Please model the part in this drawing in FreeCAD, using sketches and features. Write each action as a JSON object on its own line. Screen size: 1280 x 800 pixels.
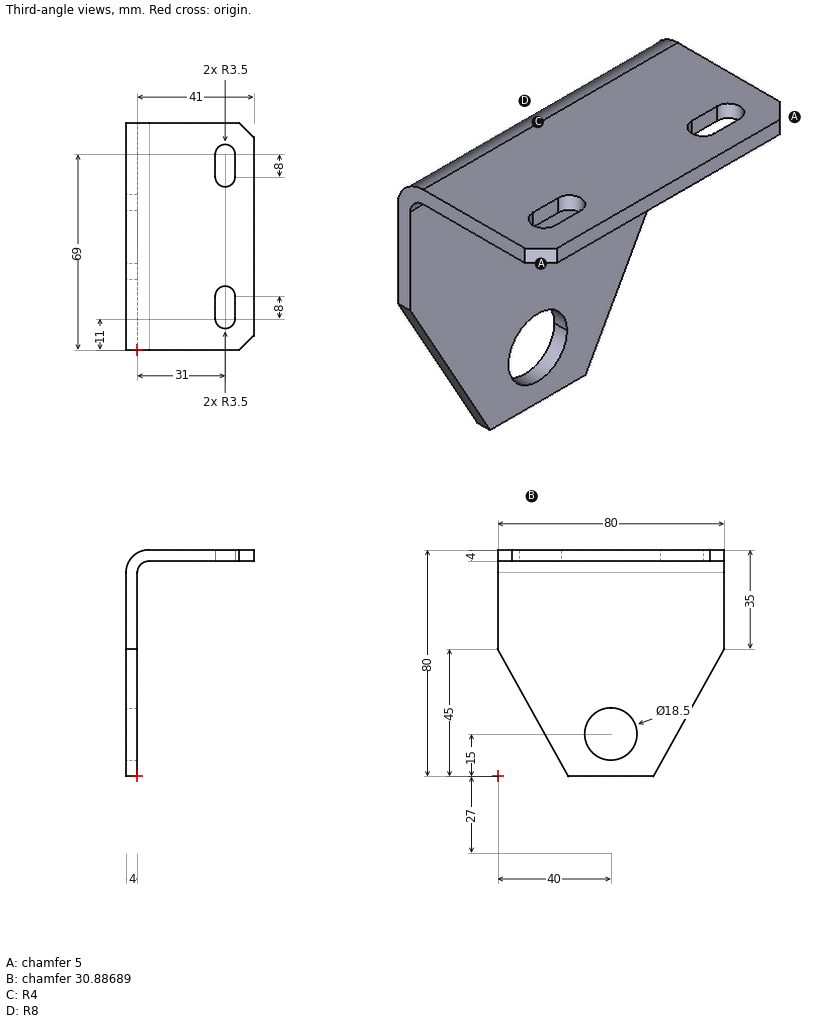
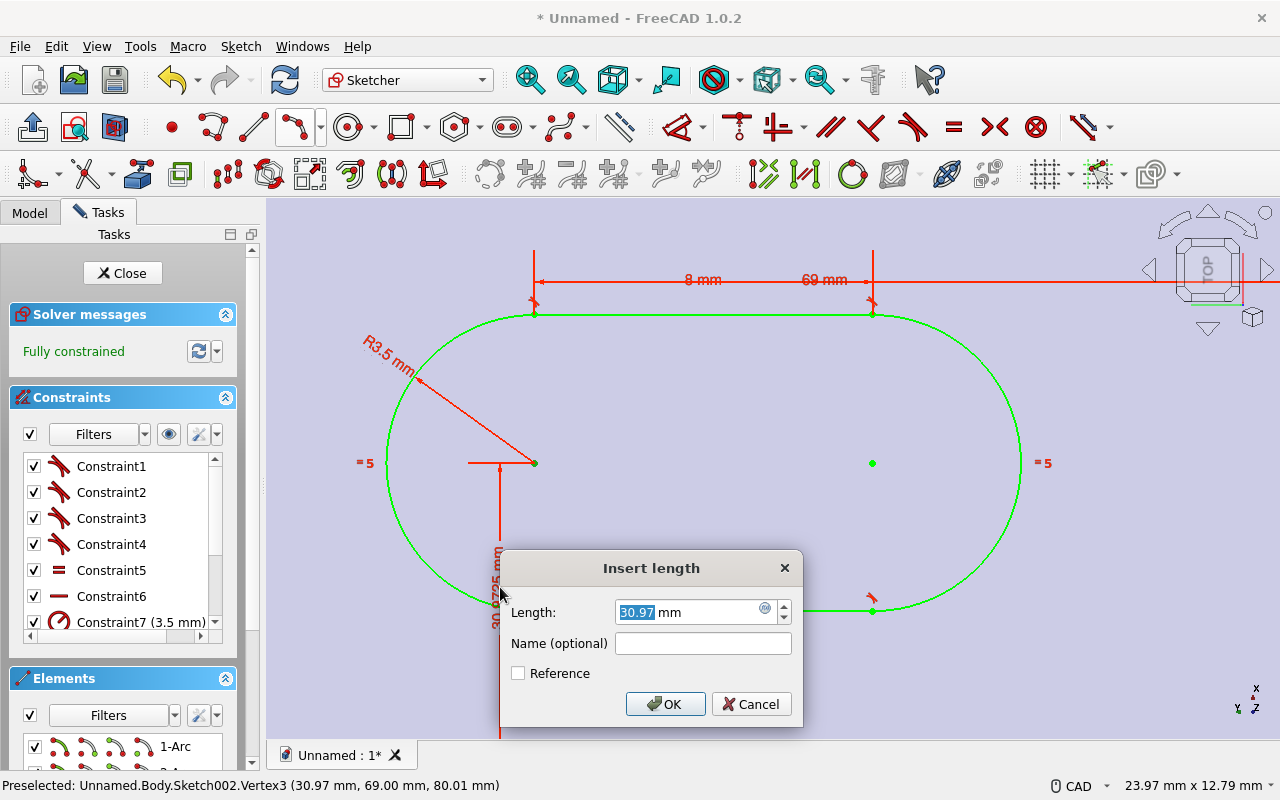
{"action": "type", "text": "31"}
{"action": "key", "text": "Return"}
{"action": "key", "text": "Escape"}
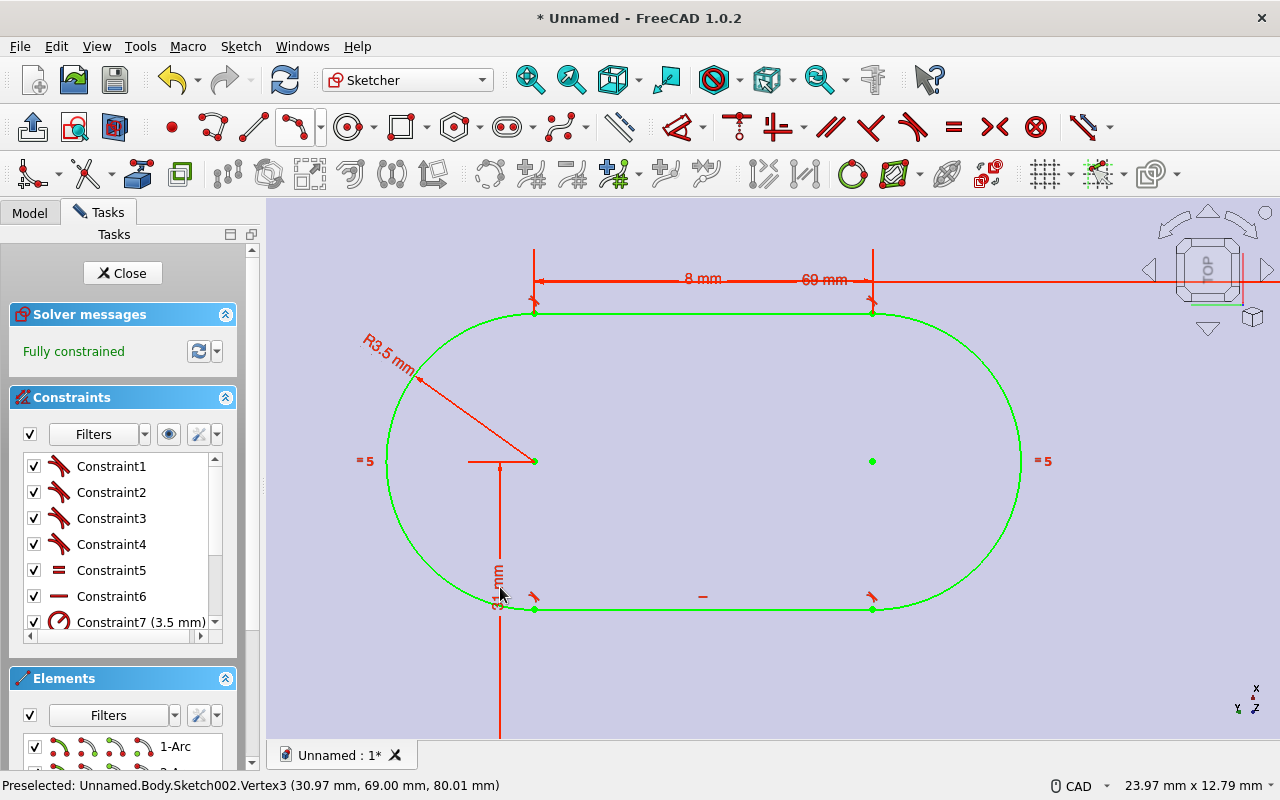
{"action": "left_click", "coordinate": [123, 273]}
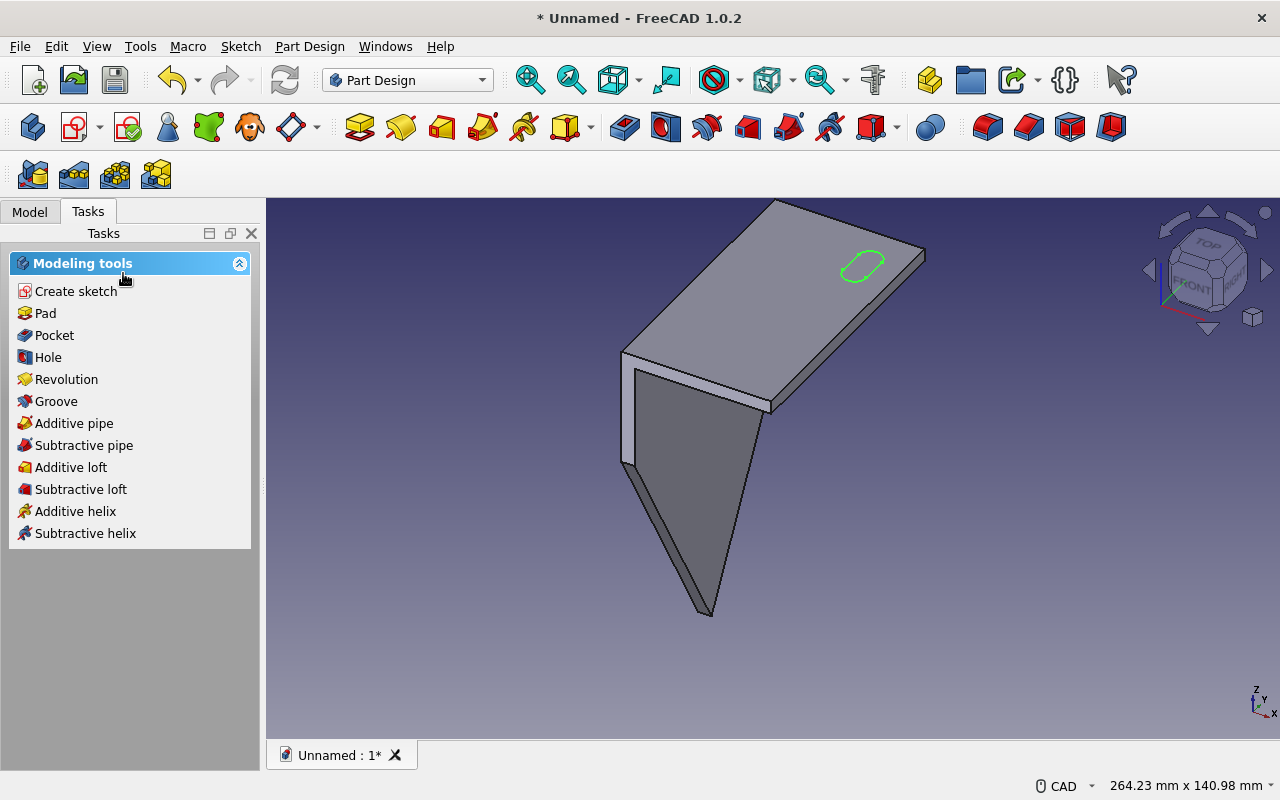
{"action": "left_click", "coordinate": [625, 128]}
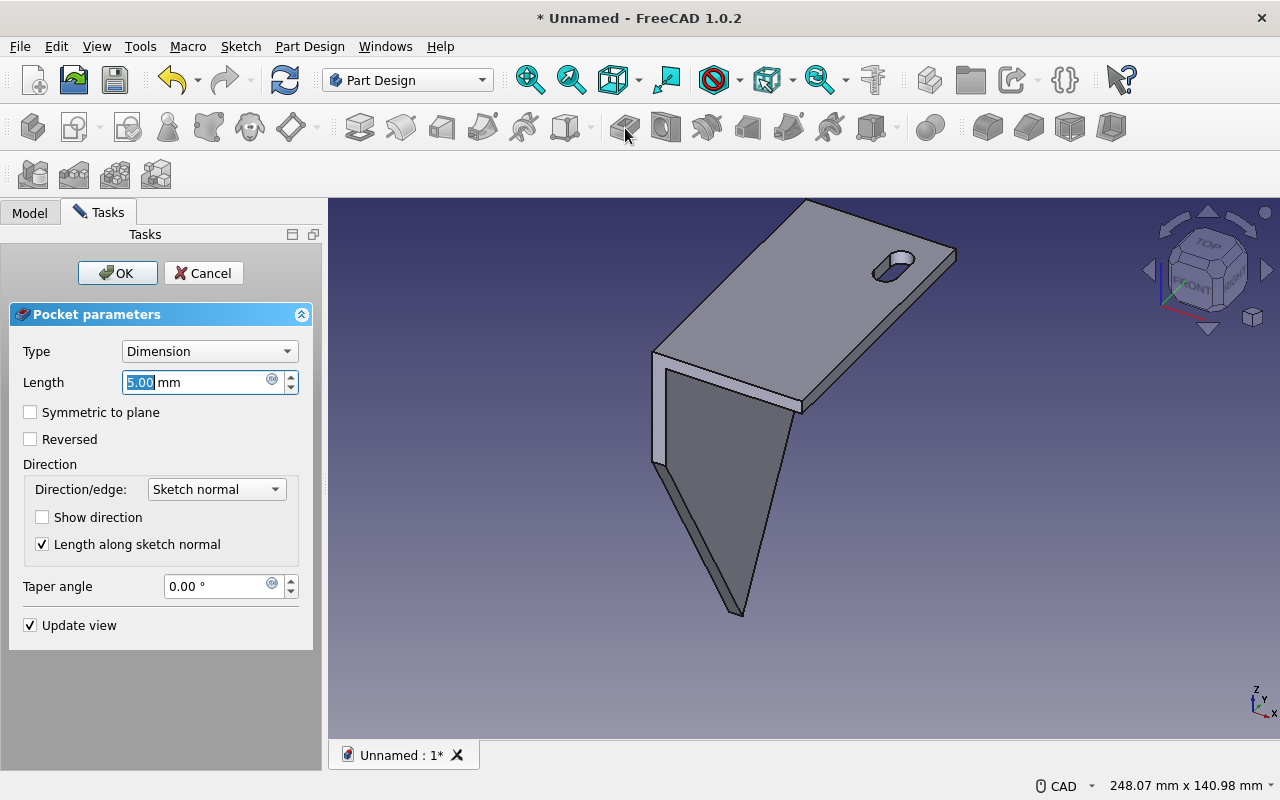
{"action": "left_click", "coordinate": [210, 352]}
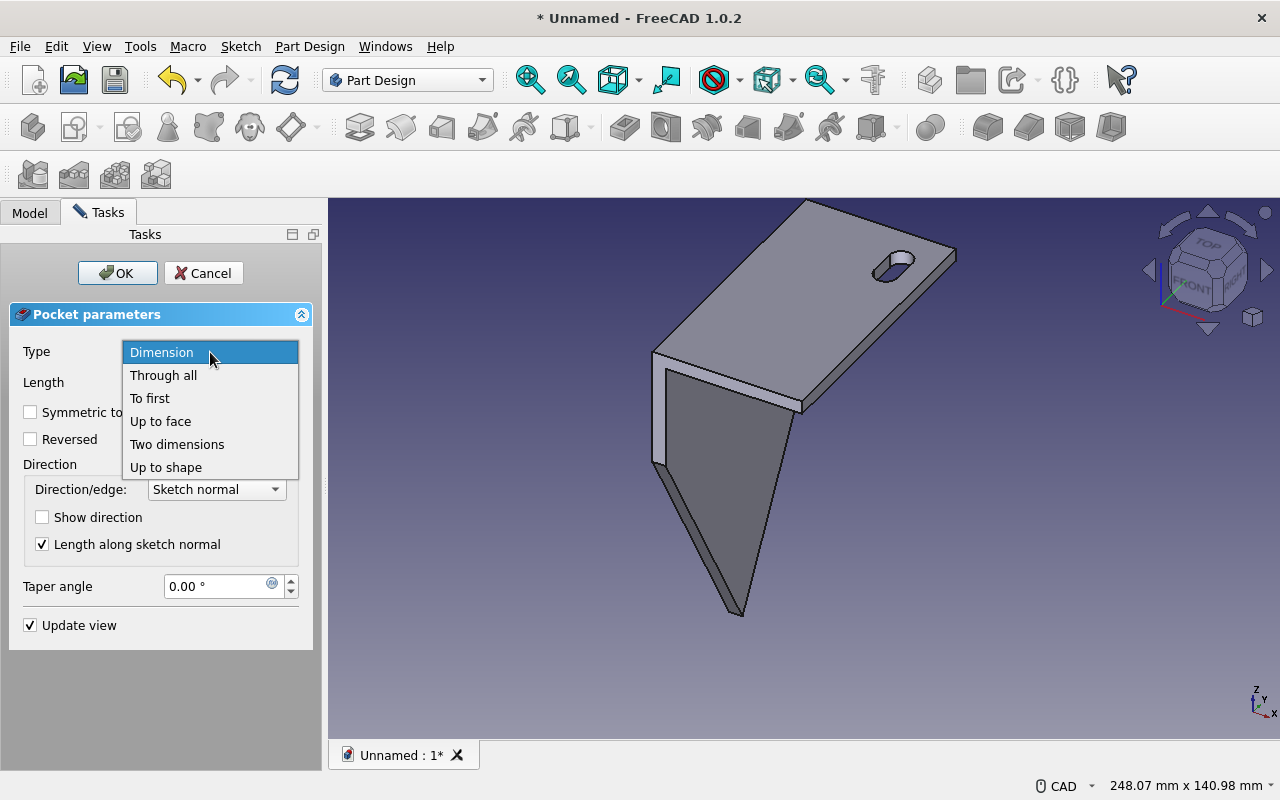
{"action": "left_click", "coordinate": [208, 376]}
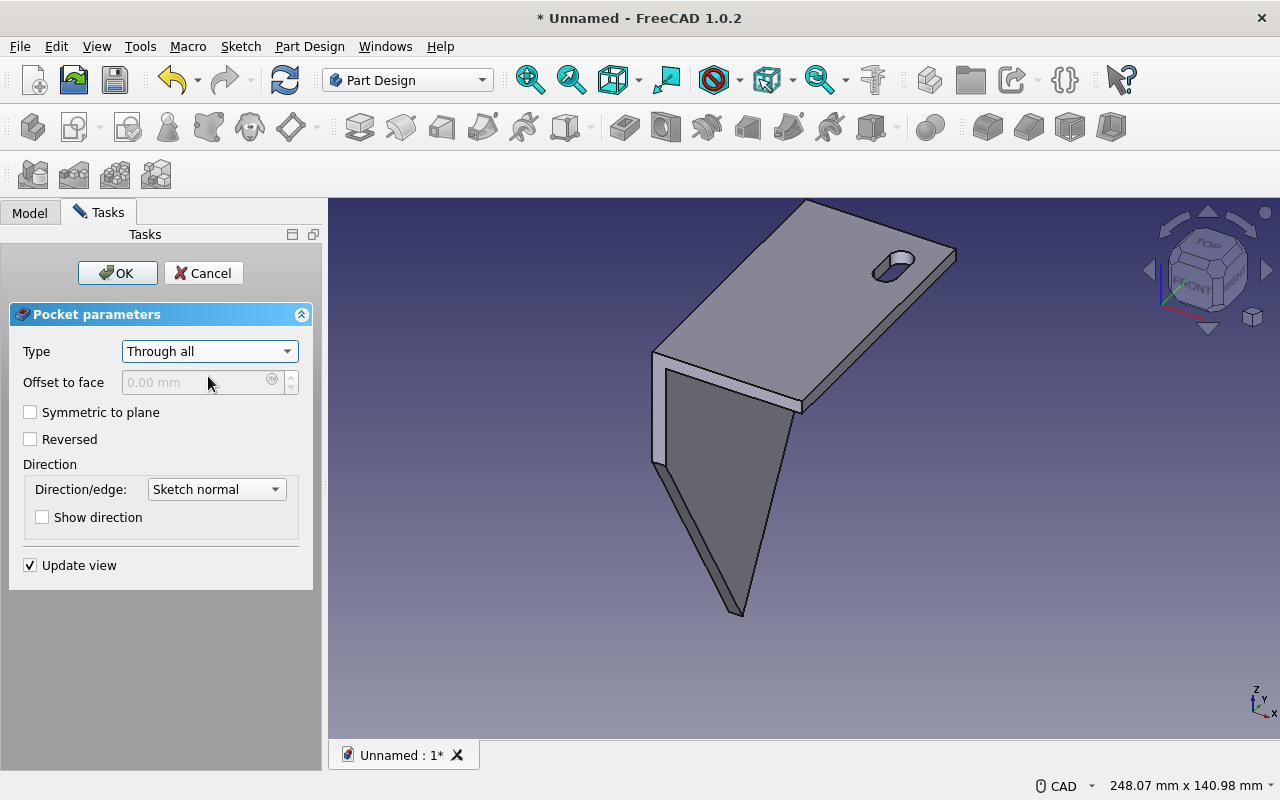
{"action": "left_click", "coordinate": [118, 273]}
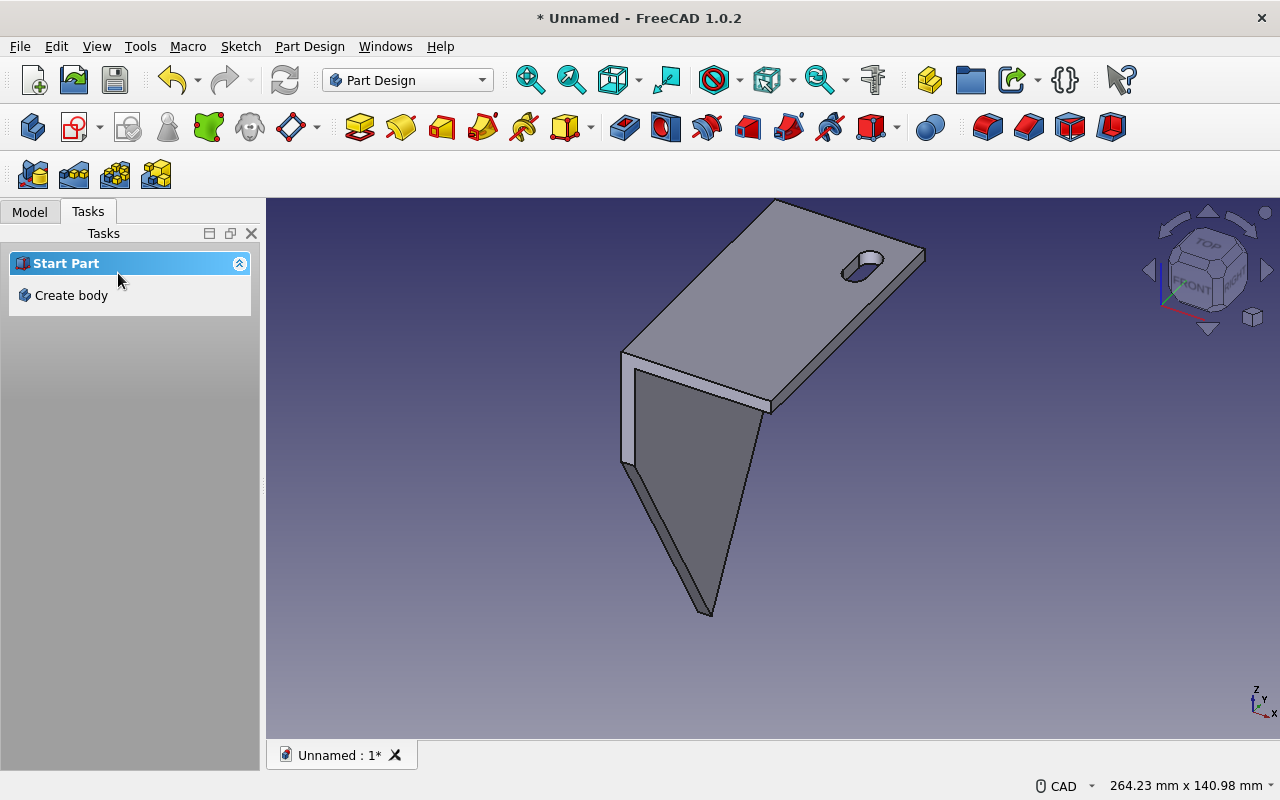
{"action": "key", "text": "5"}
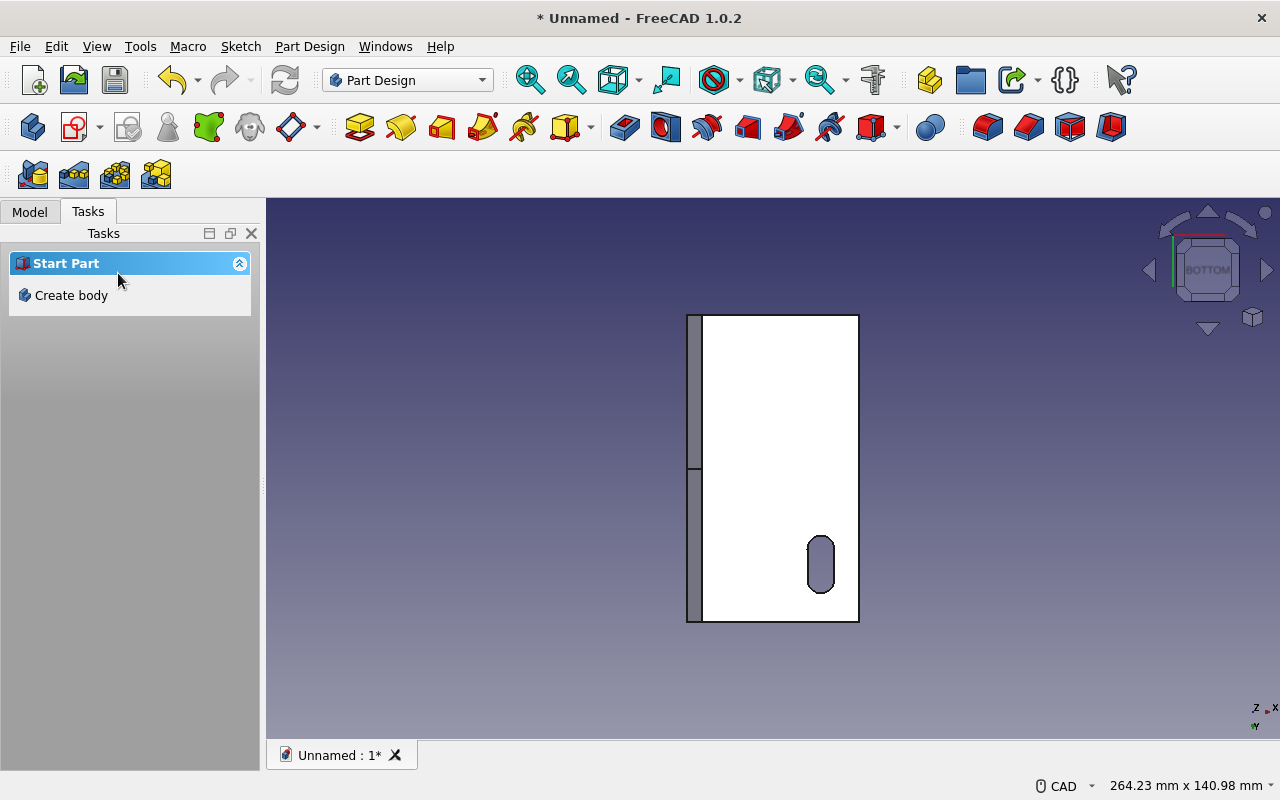
{"action": "left_click", "coordinate": [781, 424]}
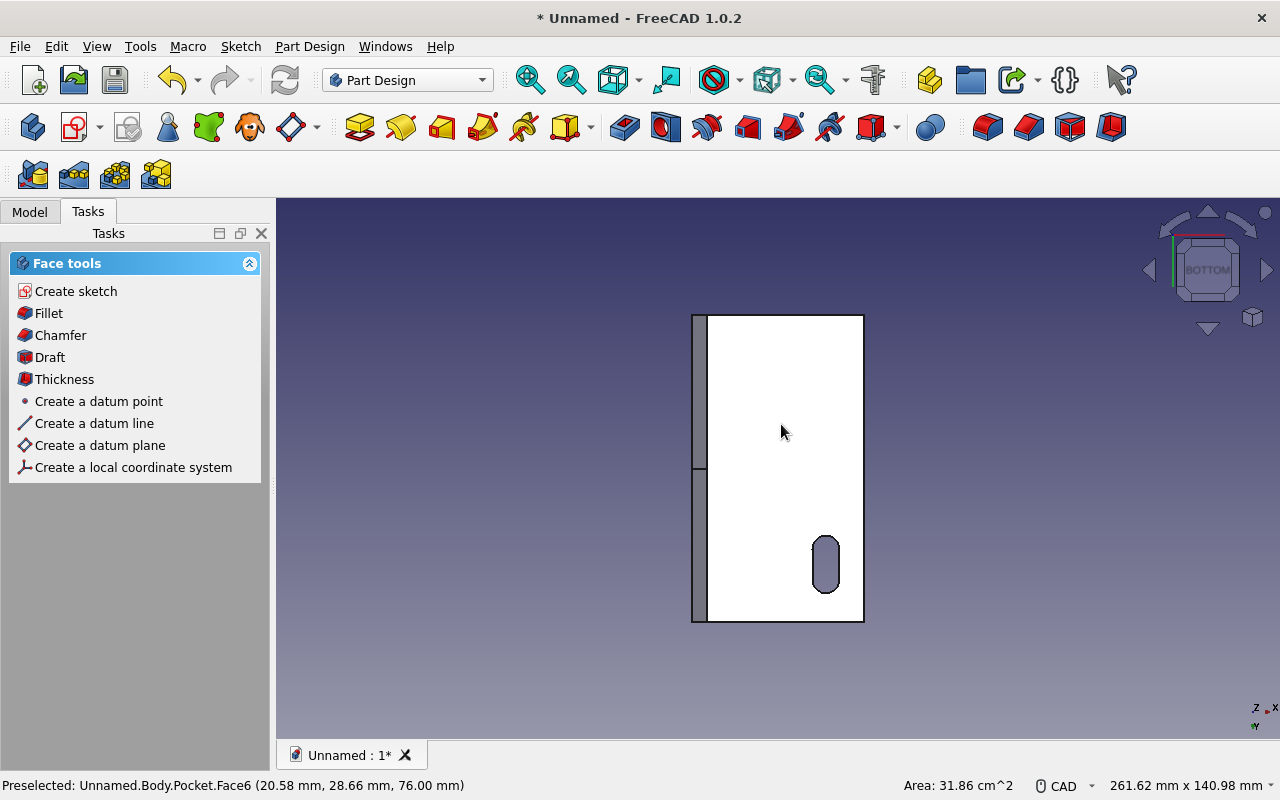
{"action": "left_click", "coordinate": [74, 128]}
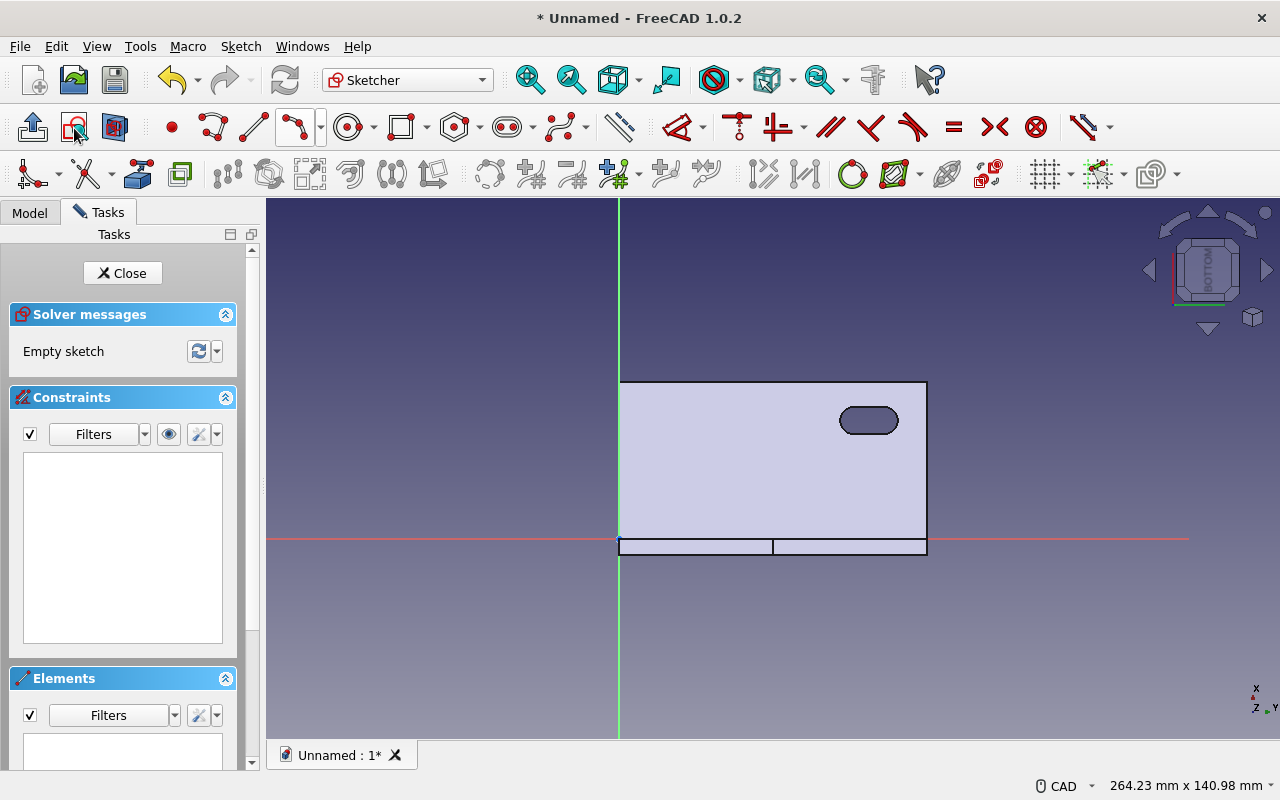
{"action": "left_click", "coordinate": [115, 128]}